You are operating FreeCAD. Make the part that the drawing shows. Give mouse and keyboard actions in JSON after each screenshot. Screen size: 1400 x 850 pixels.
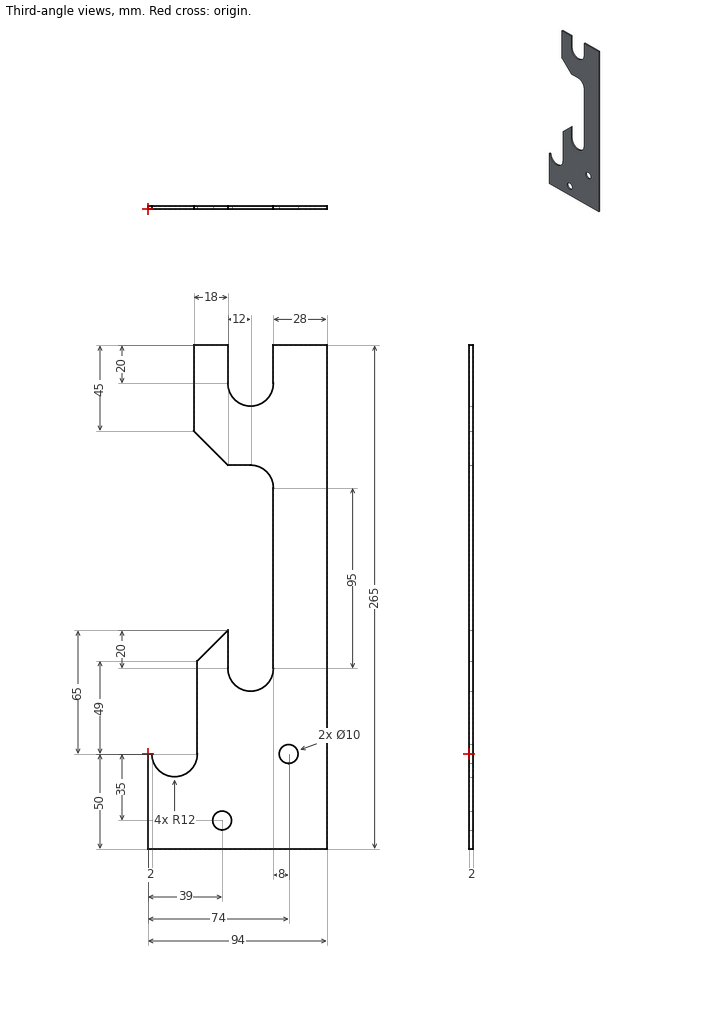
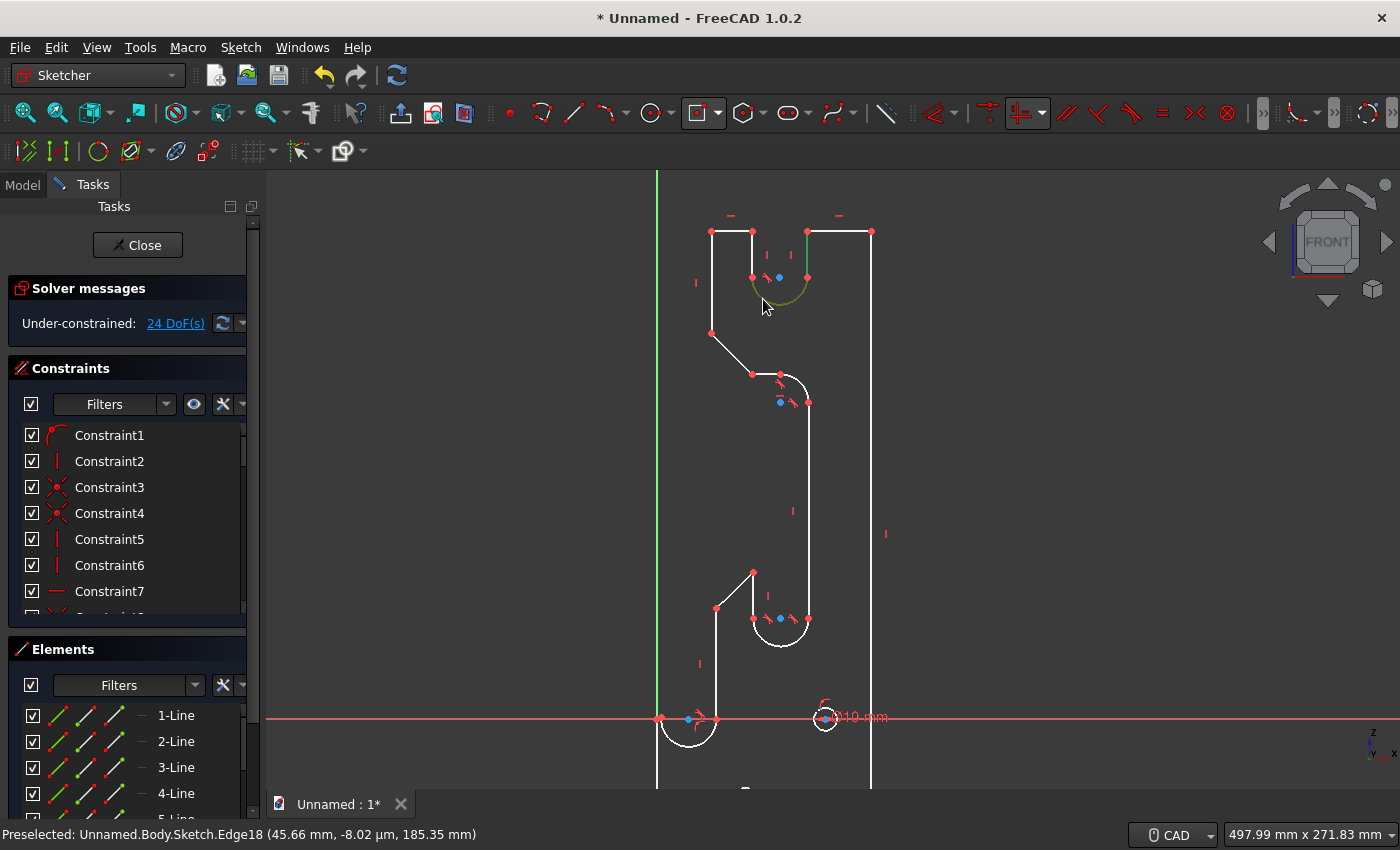
{"action": "key", "text": "t"}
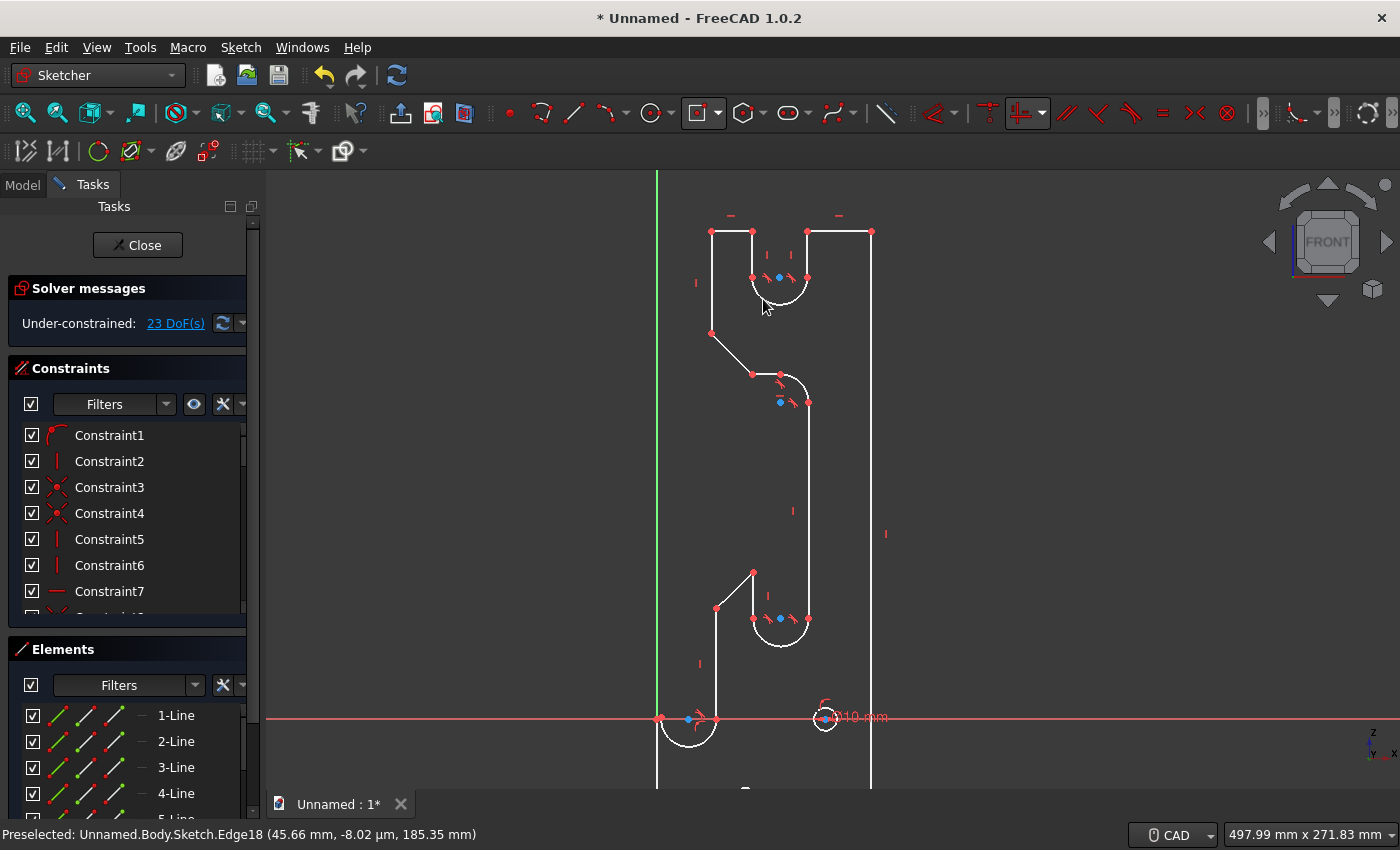
{"action": "scroll", "coordinate": [659, 718], "scroll_direction": "up", "scroll_amount": 10}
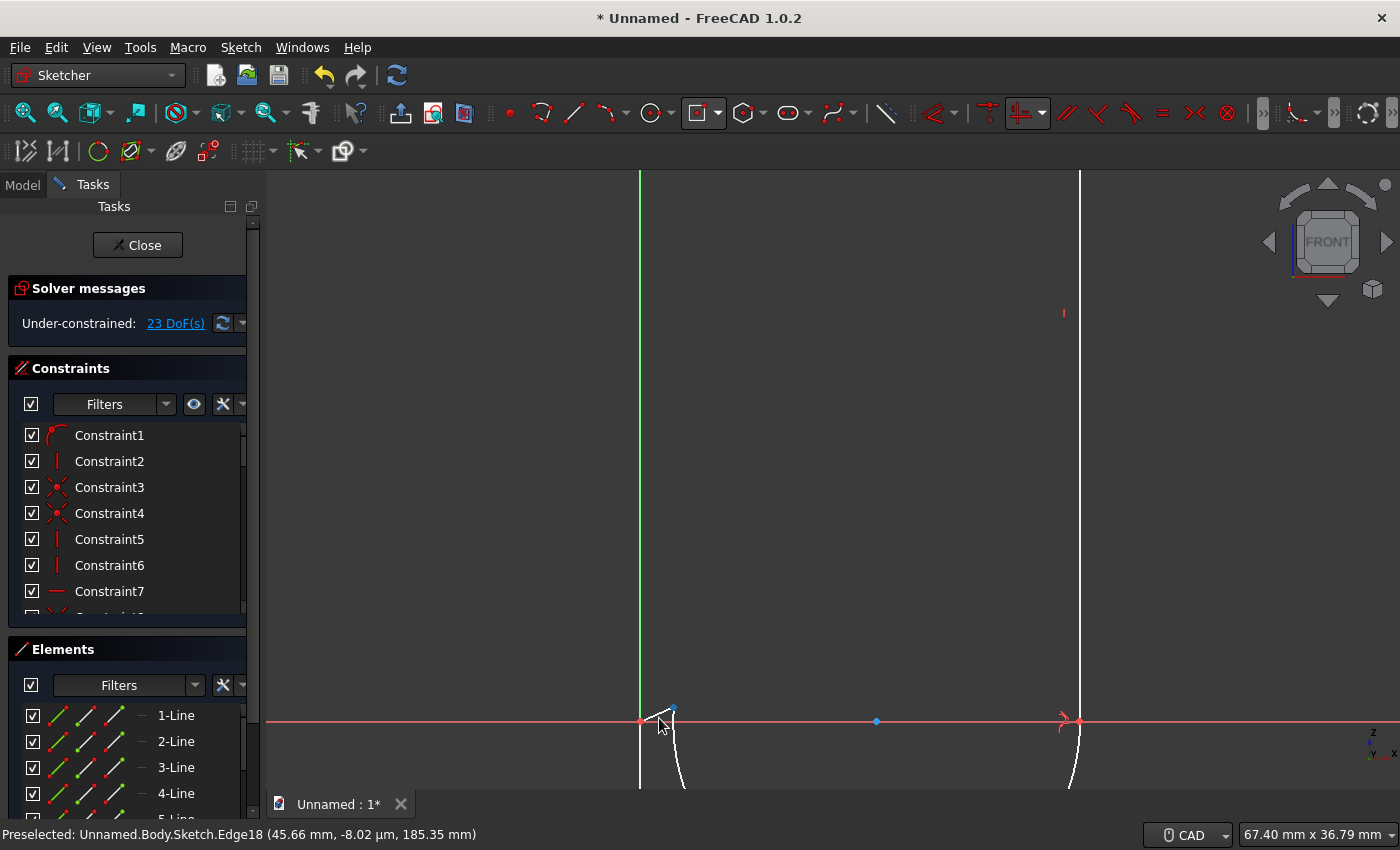
{"action": "left_click", "coordinate": [657, 715]}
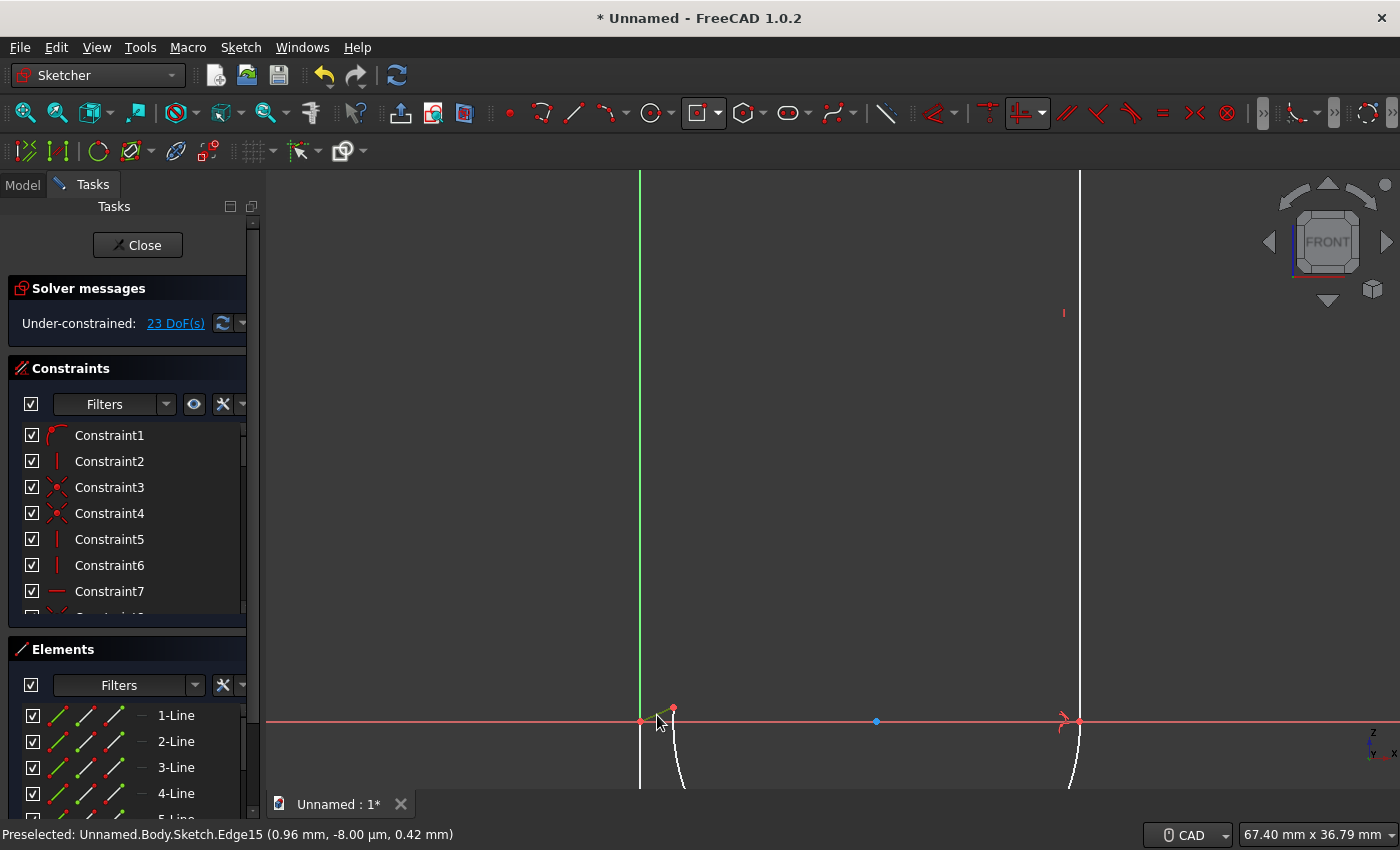
{"action": "left_click", "coordinate": [1044, 114]}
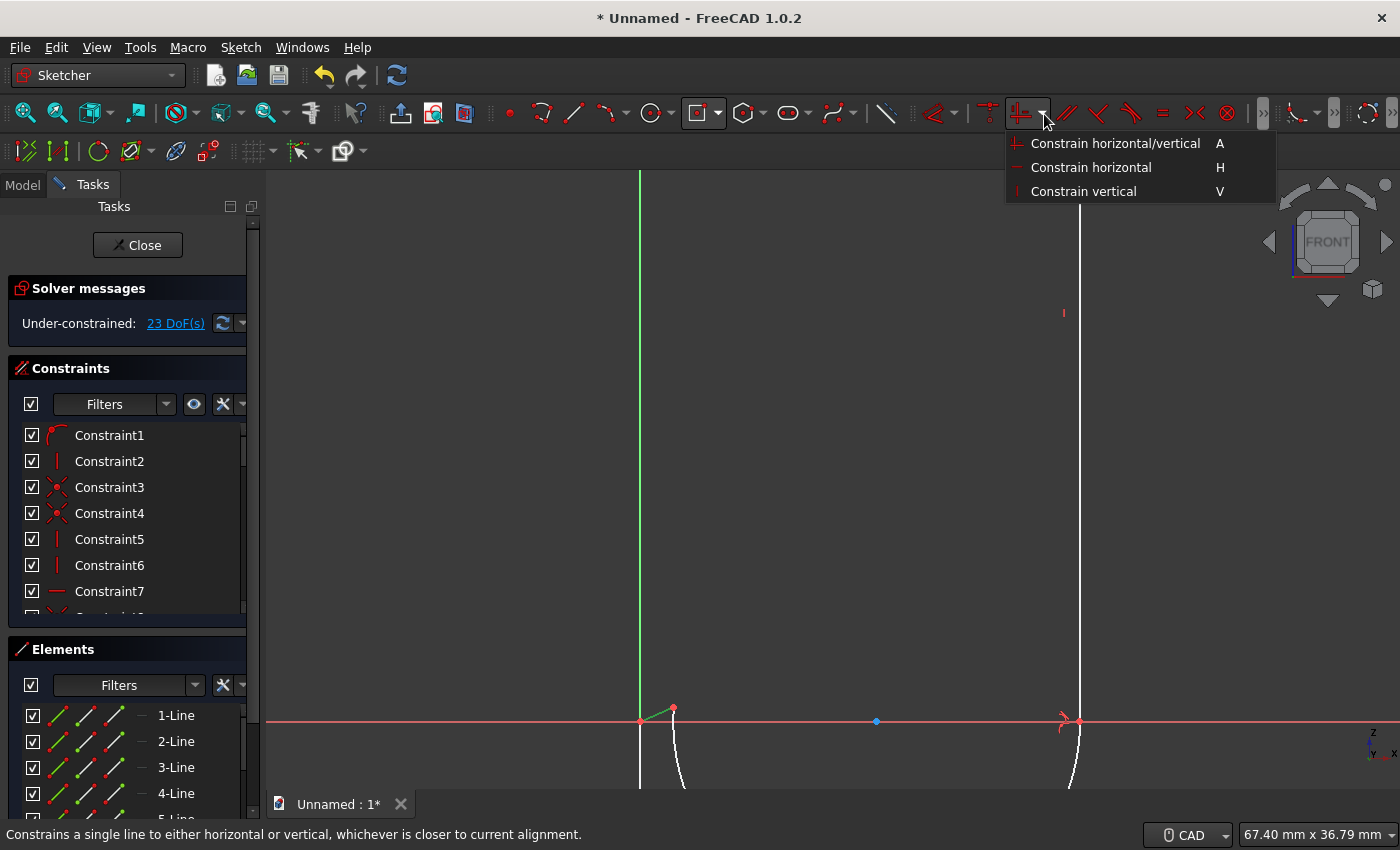
{"action": "left_click", "coordinate": [1141, 167]}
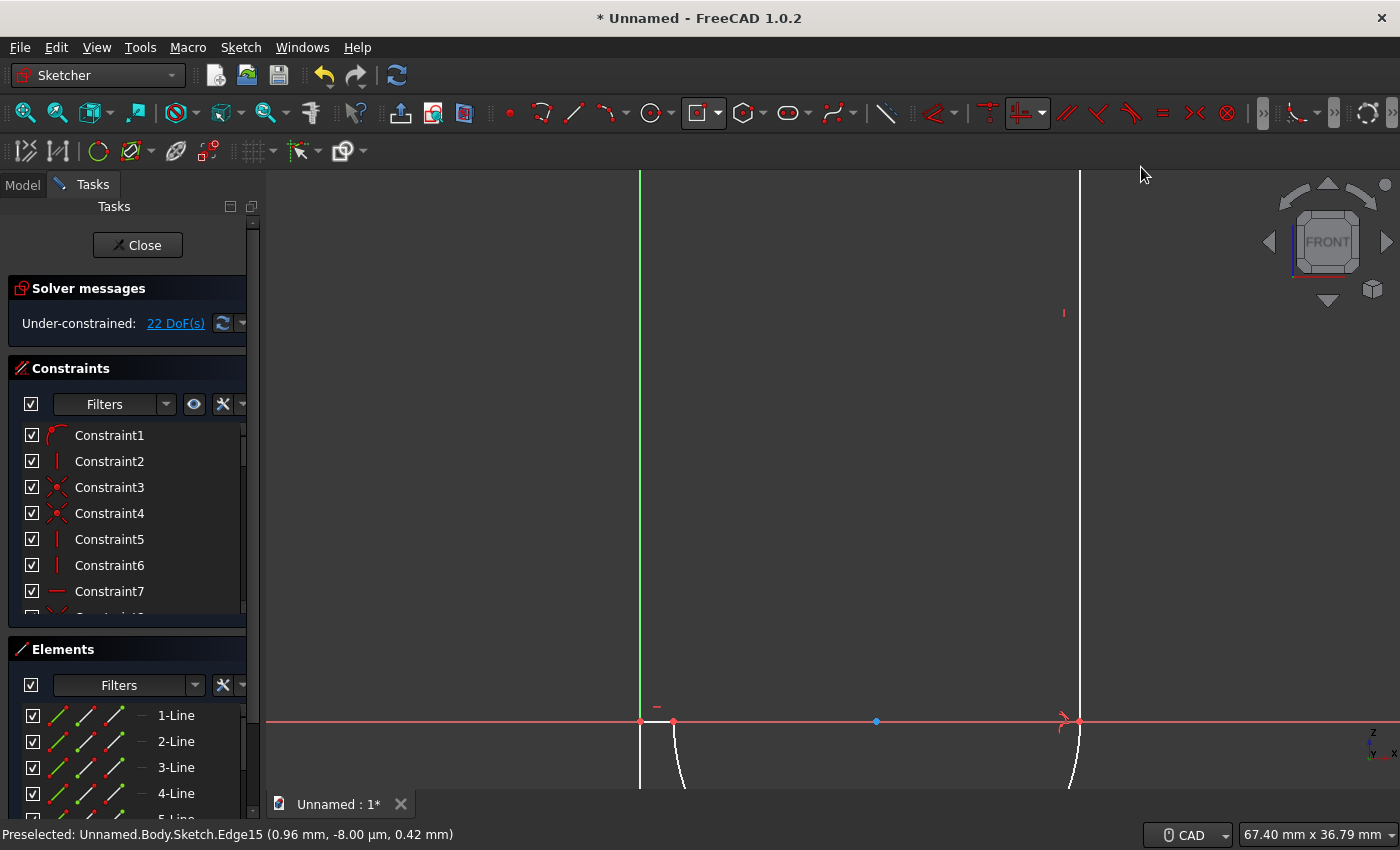
{"action": "scroll", "coordinate": [698, 594], "scroll_direction": "down", "scroll_amount": 12}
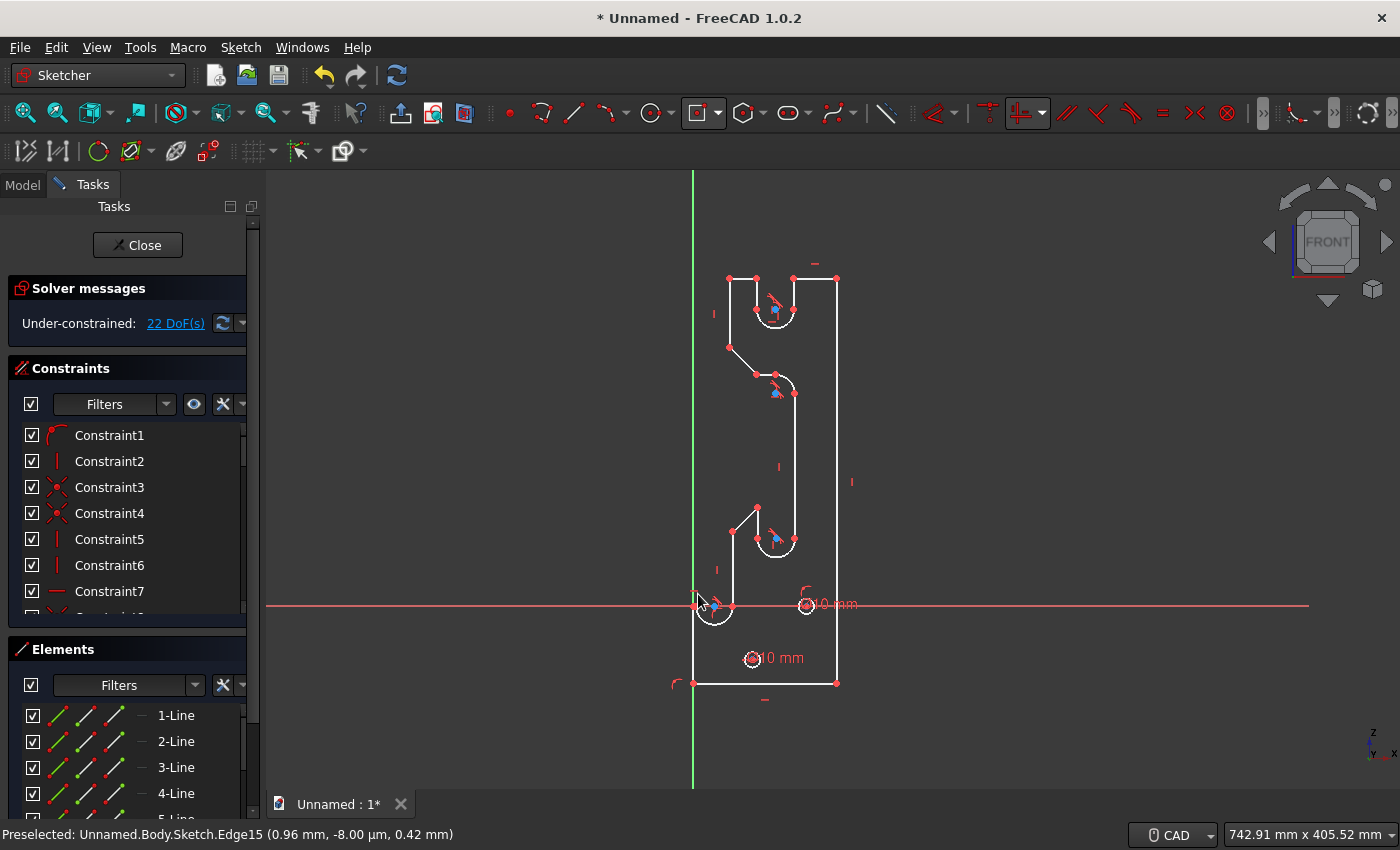
{"action": "left_click", "coordinate": [765, 554]}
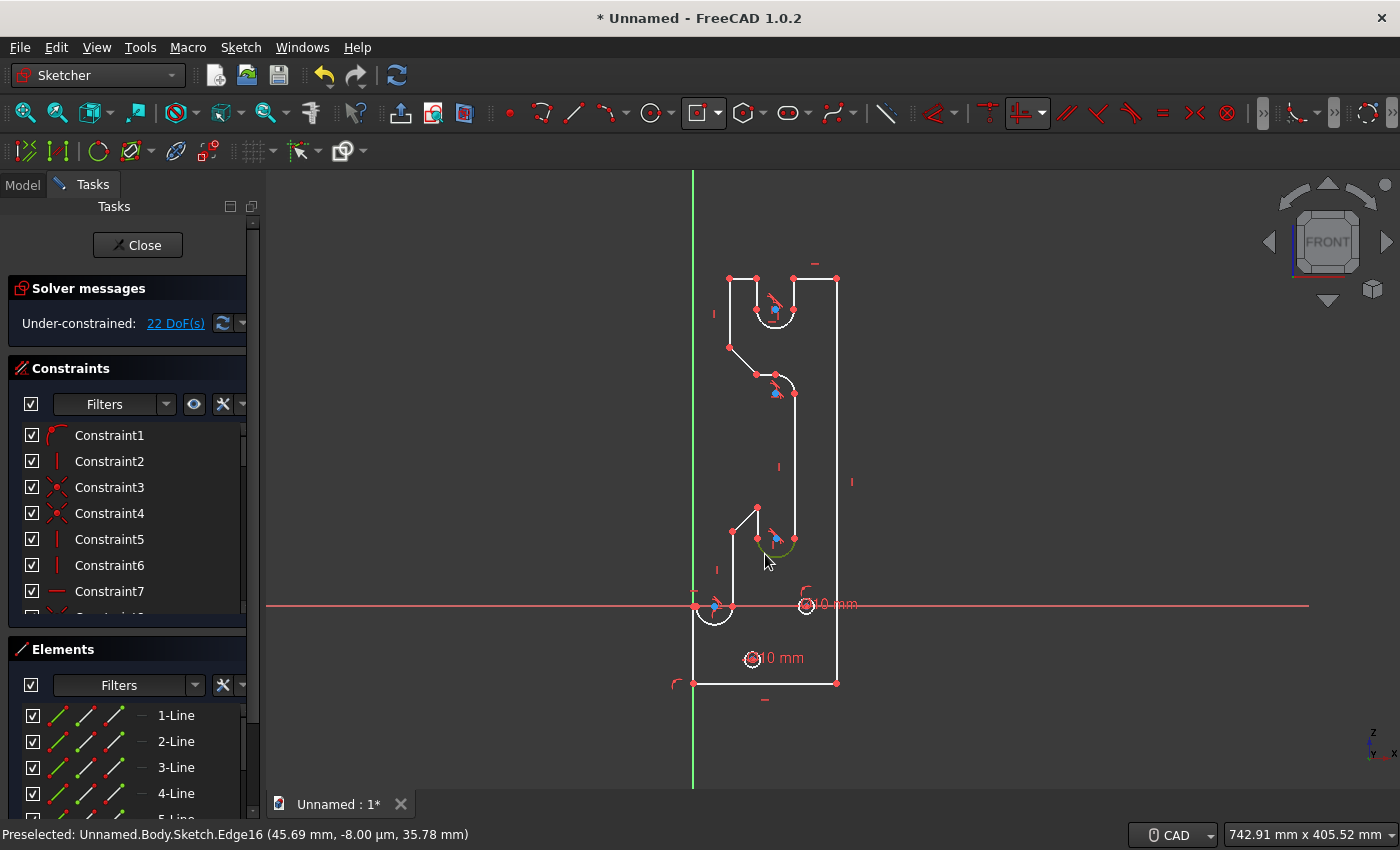
{"action": "left_click", "coordinate": [789, 381]}